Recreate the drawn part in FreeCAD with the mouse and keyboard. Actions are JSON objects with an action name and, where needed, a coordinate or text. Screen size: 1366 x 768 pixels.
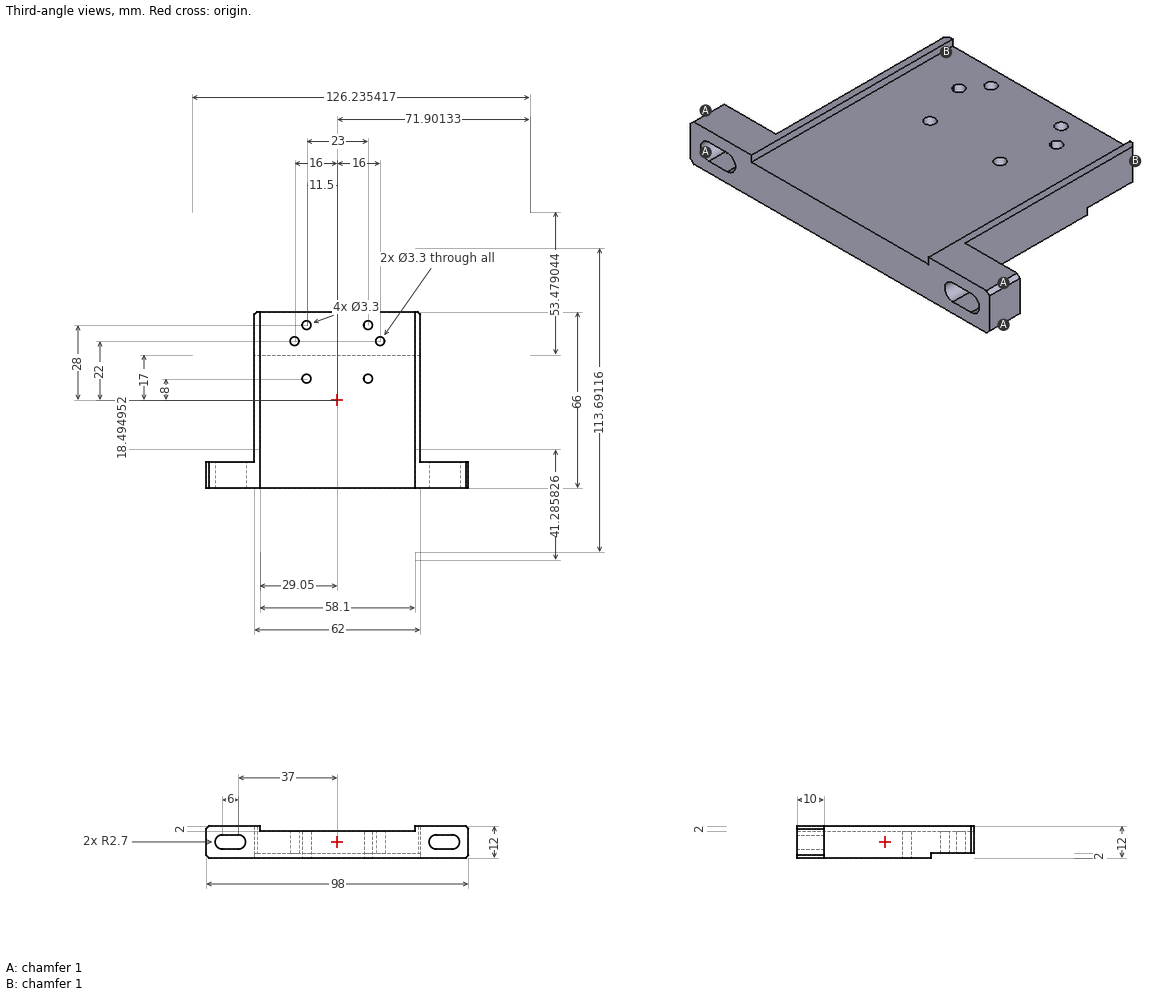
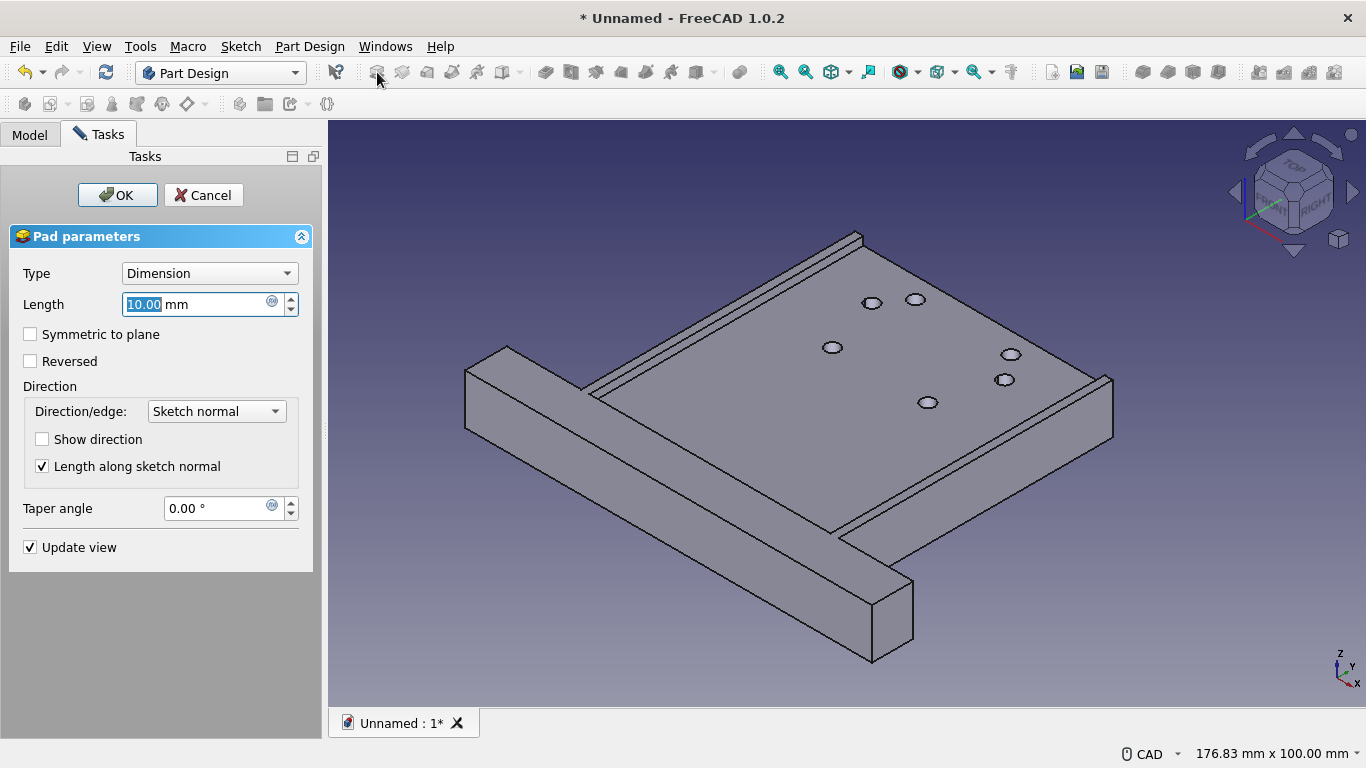
{"action": "type", "text": "10"}
{"action": "key", "text": "Tab"}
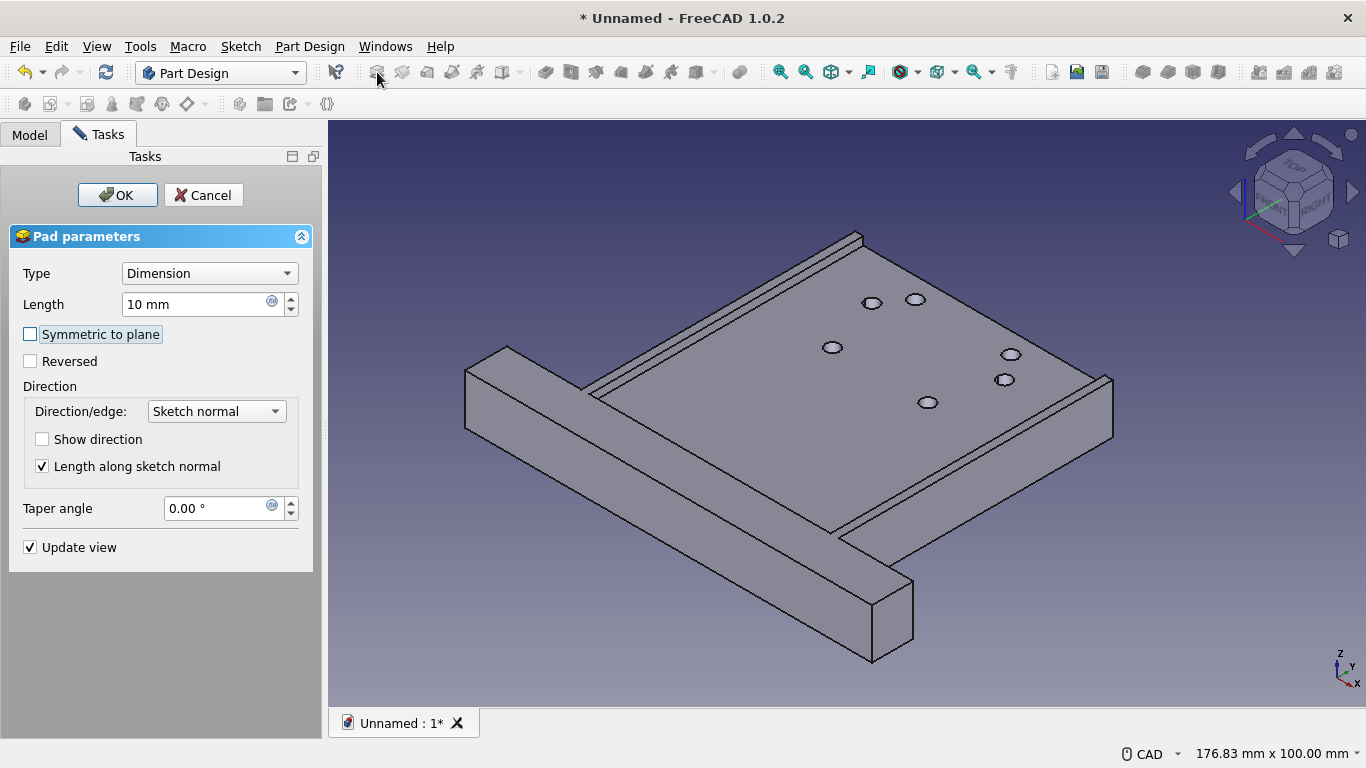
{"action": "left_click", "coordinate": [31, 361]}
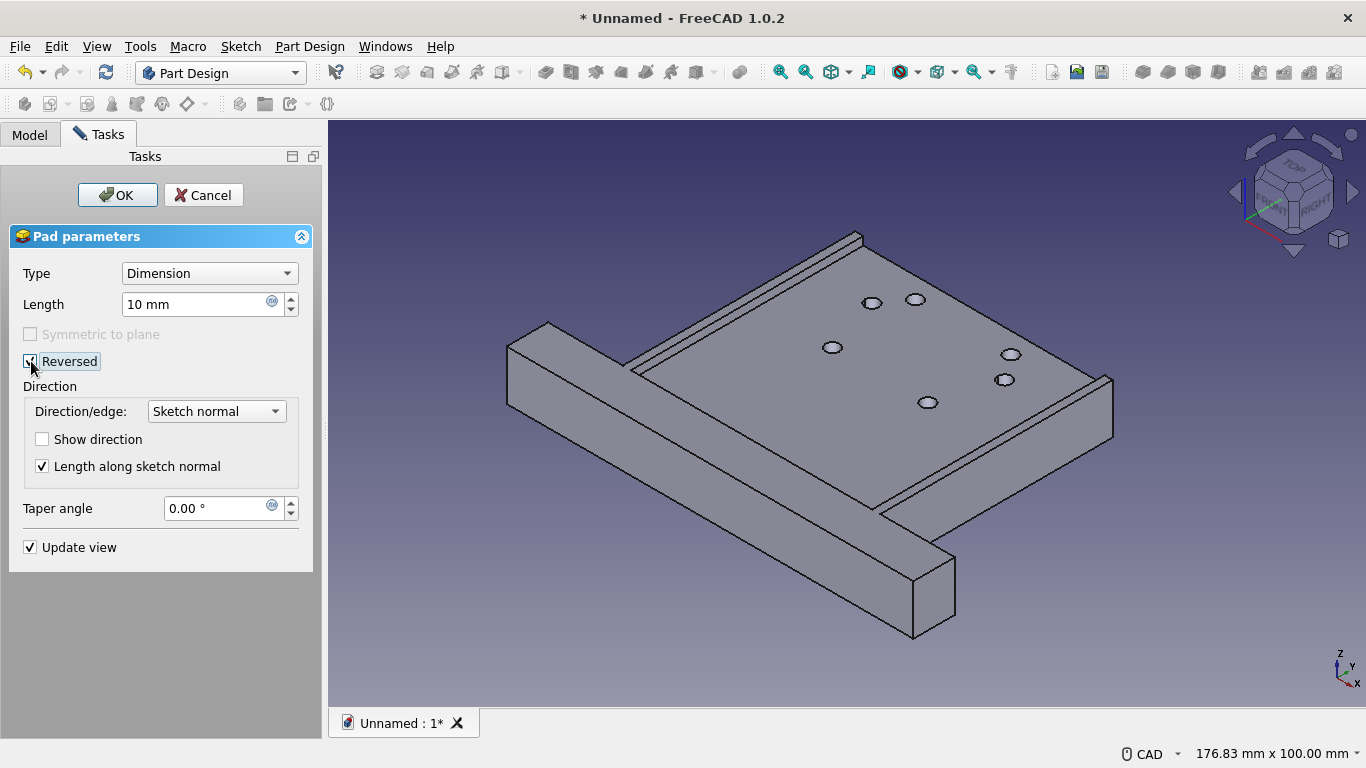
{"action": "left_click", "coordinate": [118, 195]}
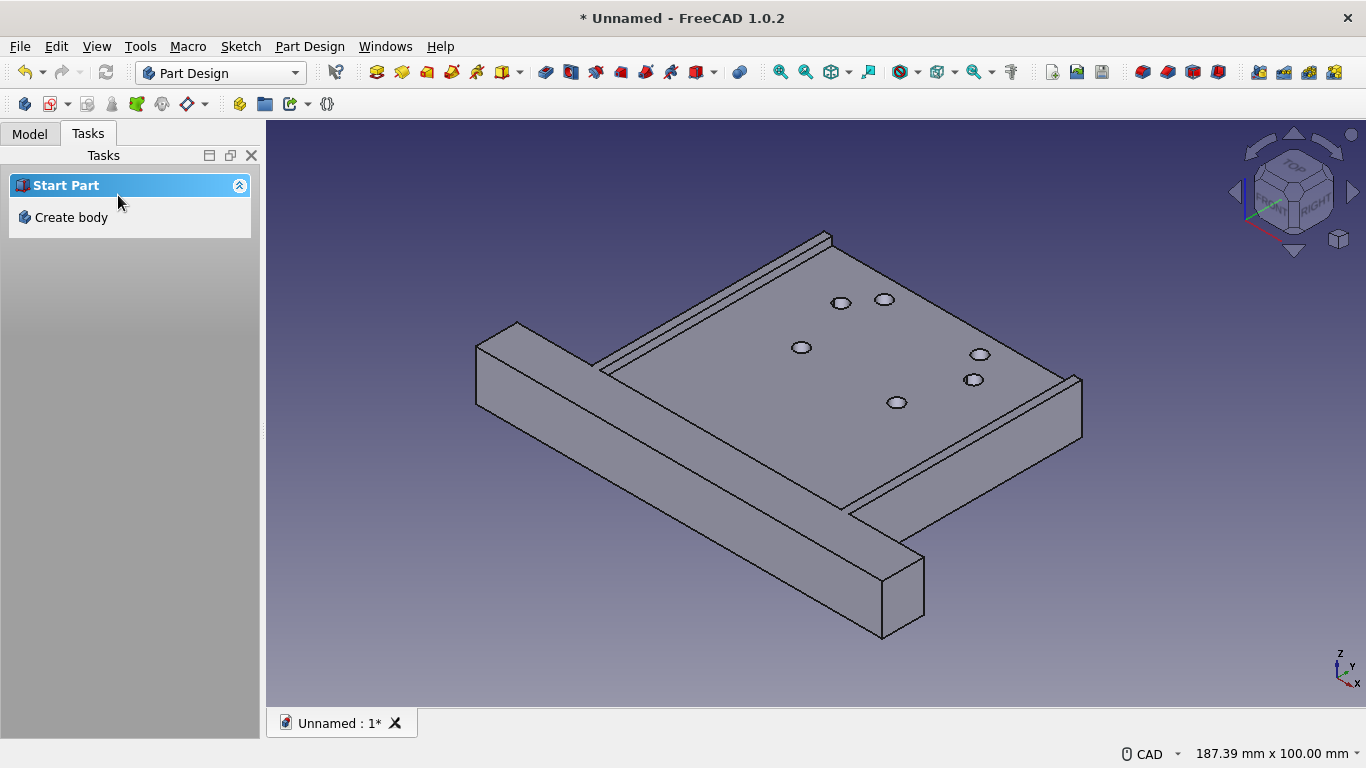
{"action": "key", "text": "4"}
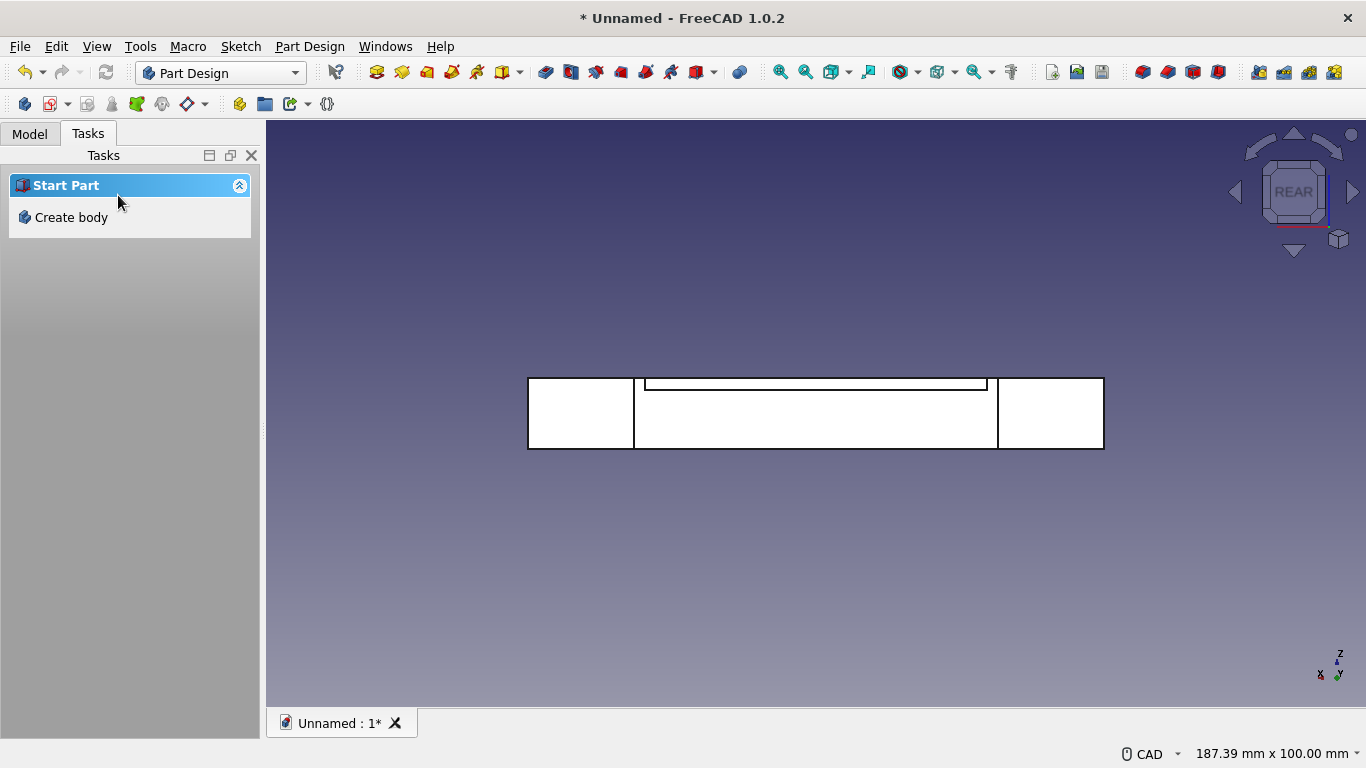
{"action": "left_click", "coordinate": [1036, 412]}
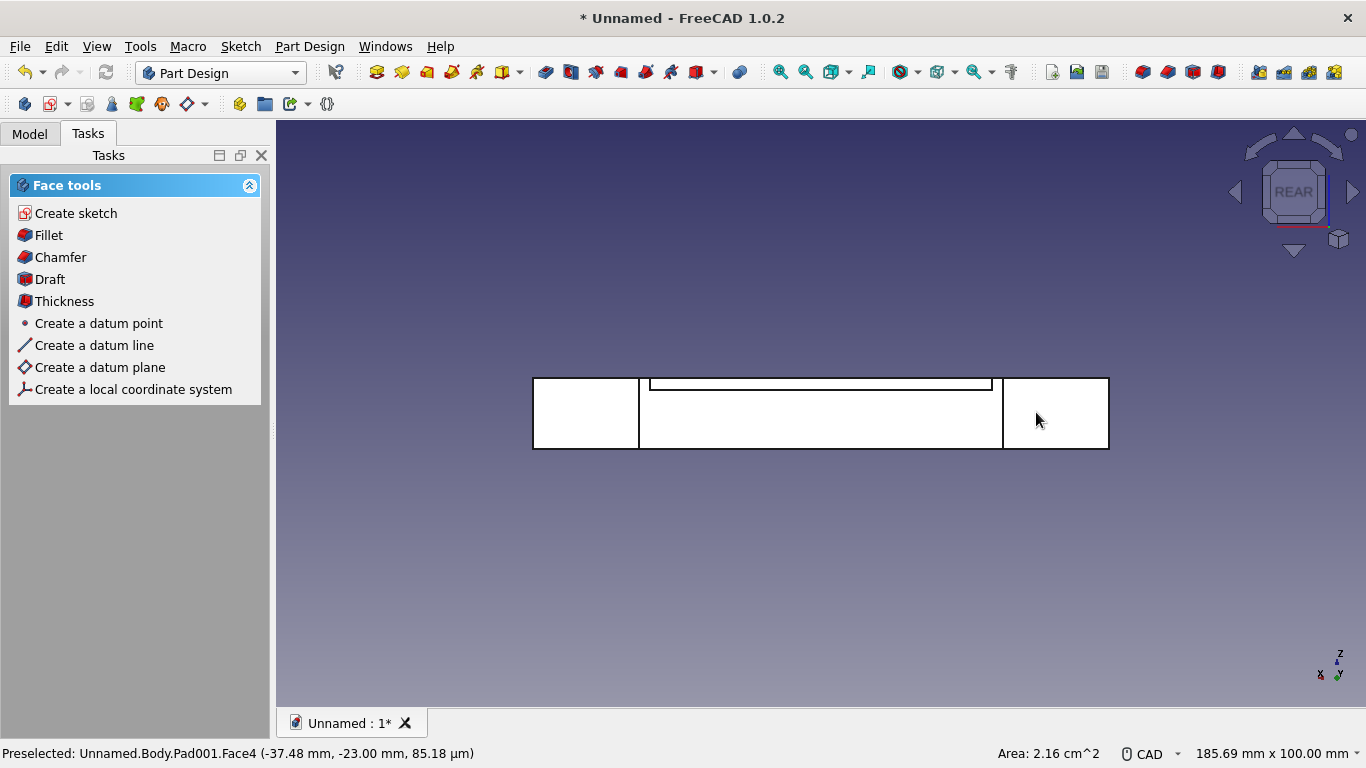
{"action": "left_click", "coordinate": [50, 104]}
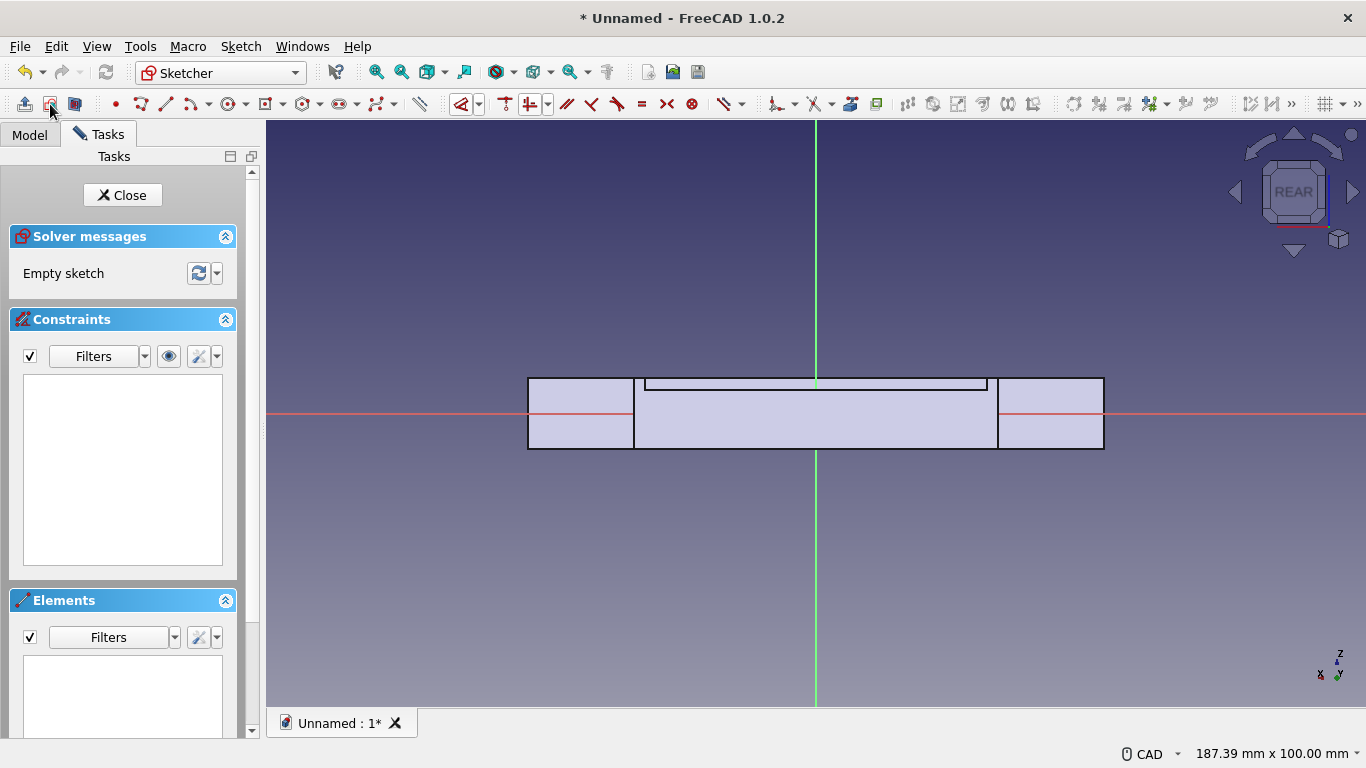
{"action": "left_click", "coordinate": [75, 104]}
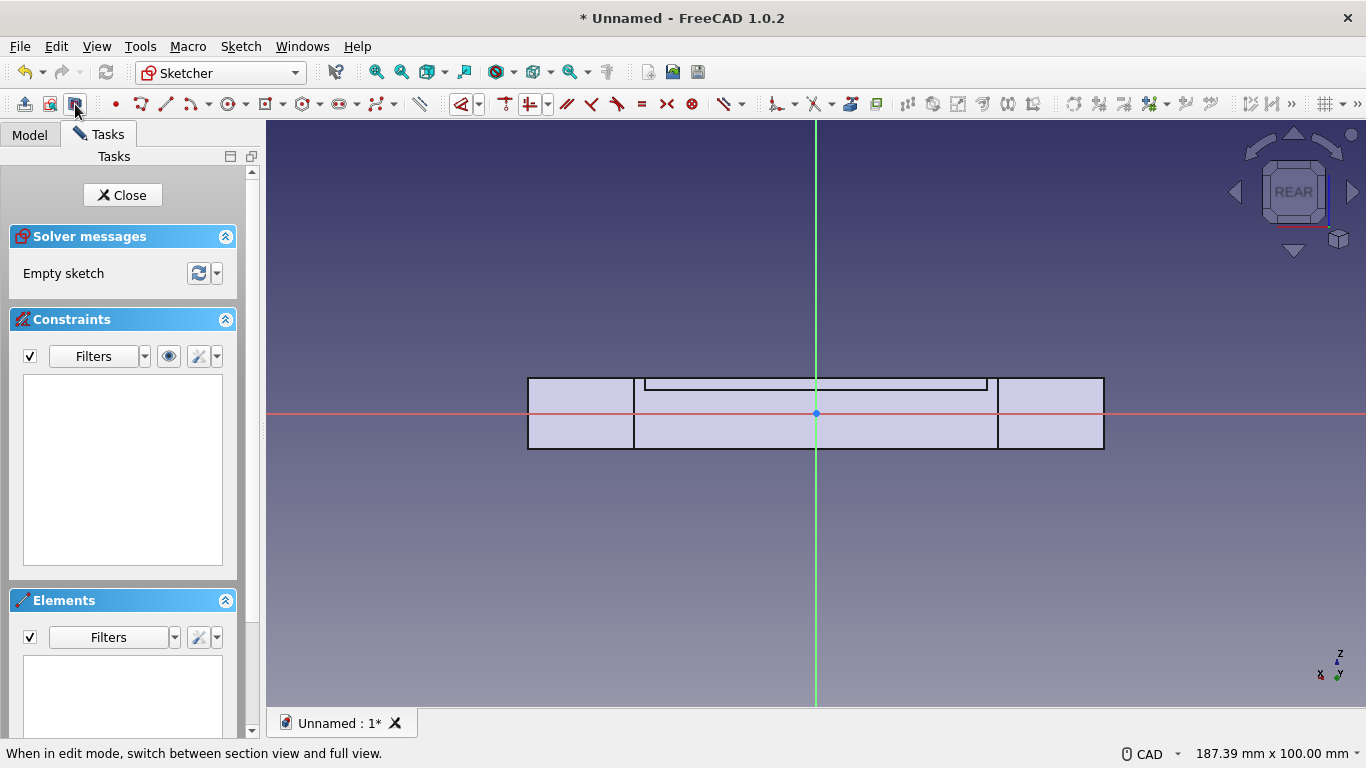
{"action": "scroll", "coordinate": [1089, 413], "scroll_direction": "up", "scroll_amount": 11}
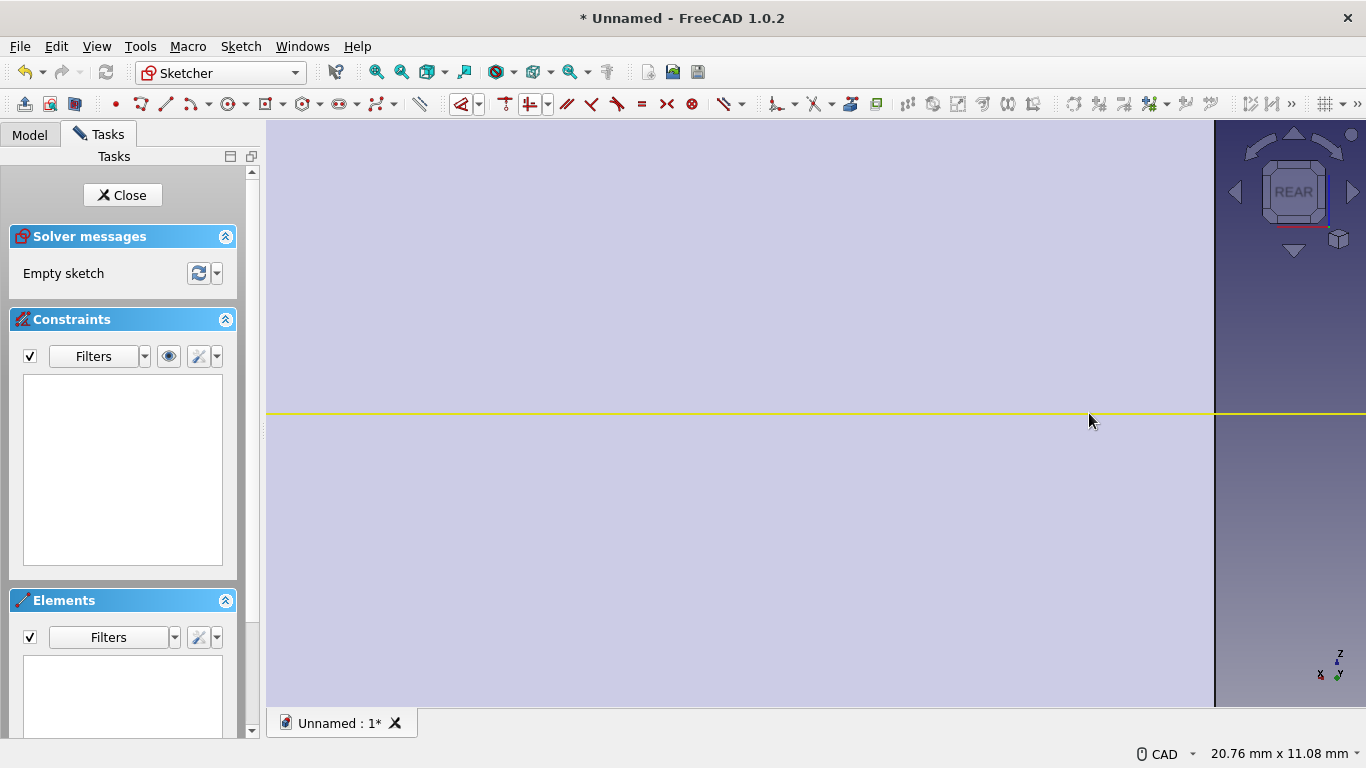
{"action": "left_click", "coordinate": [338, 104]}